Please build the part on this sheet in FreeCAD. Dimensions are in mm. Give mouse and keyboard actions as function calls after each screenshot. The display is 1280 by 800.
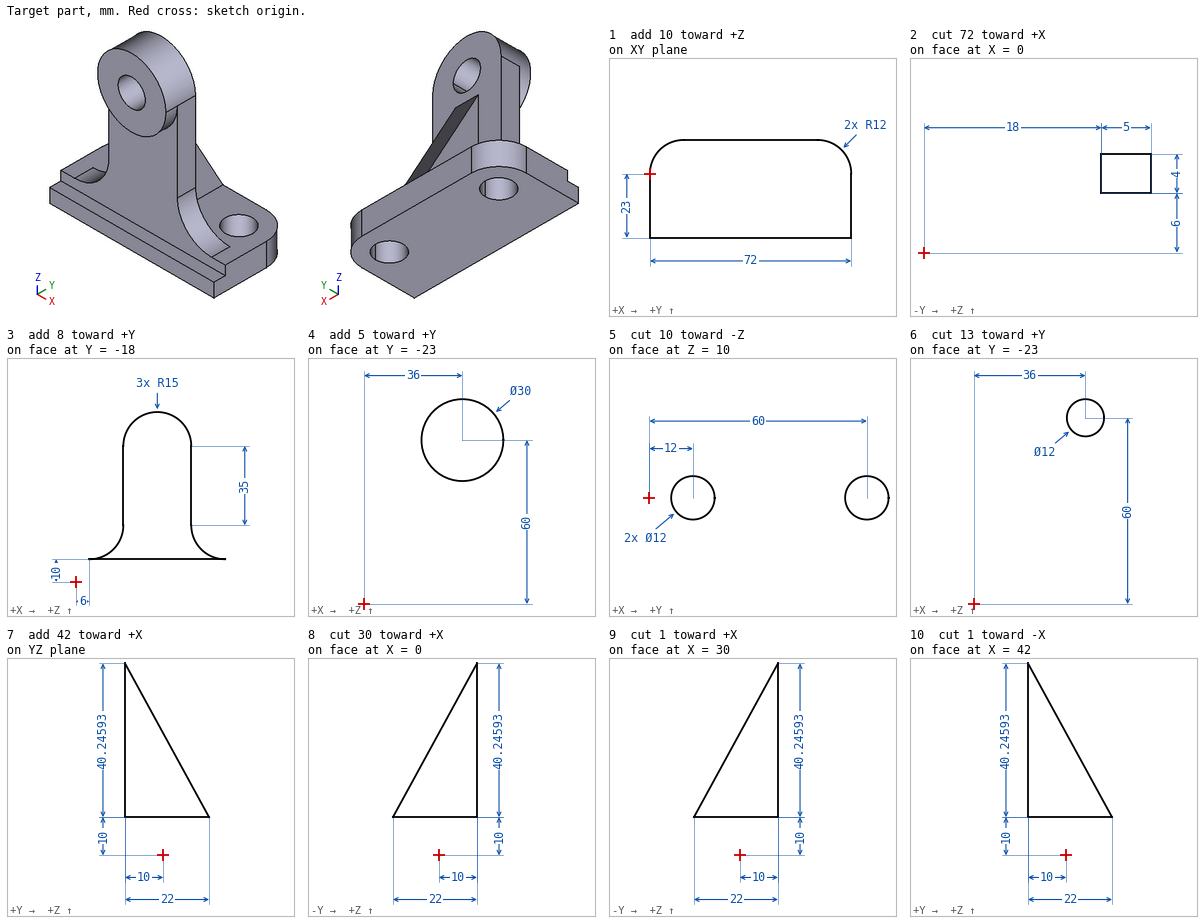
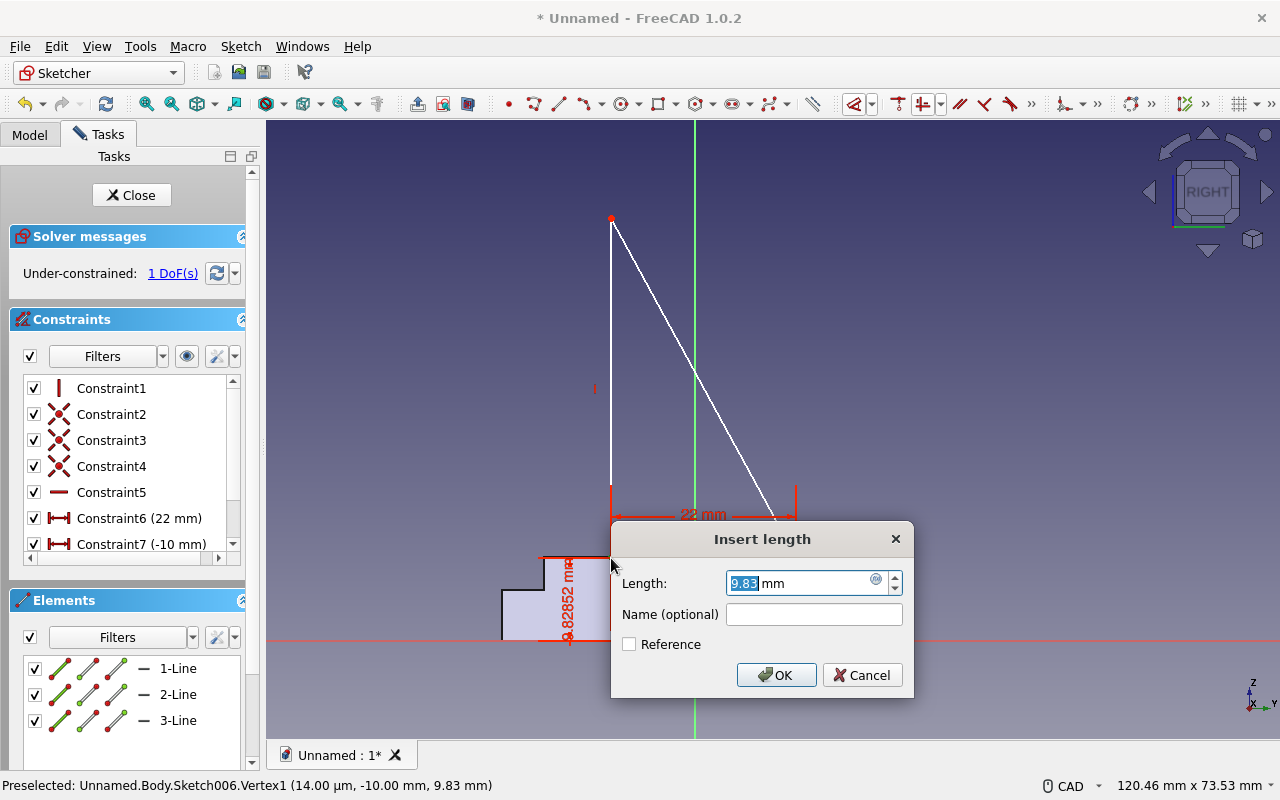
text(10)
key(Return)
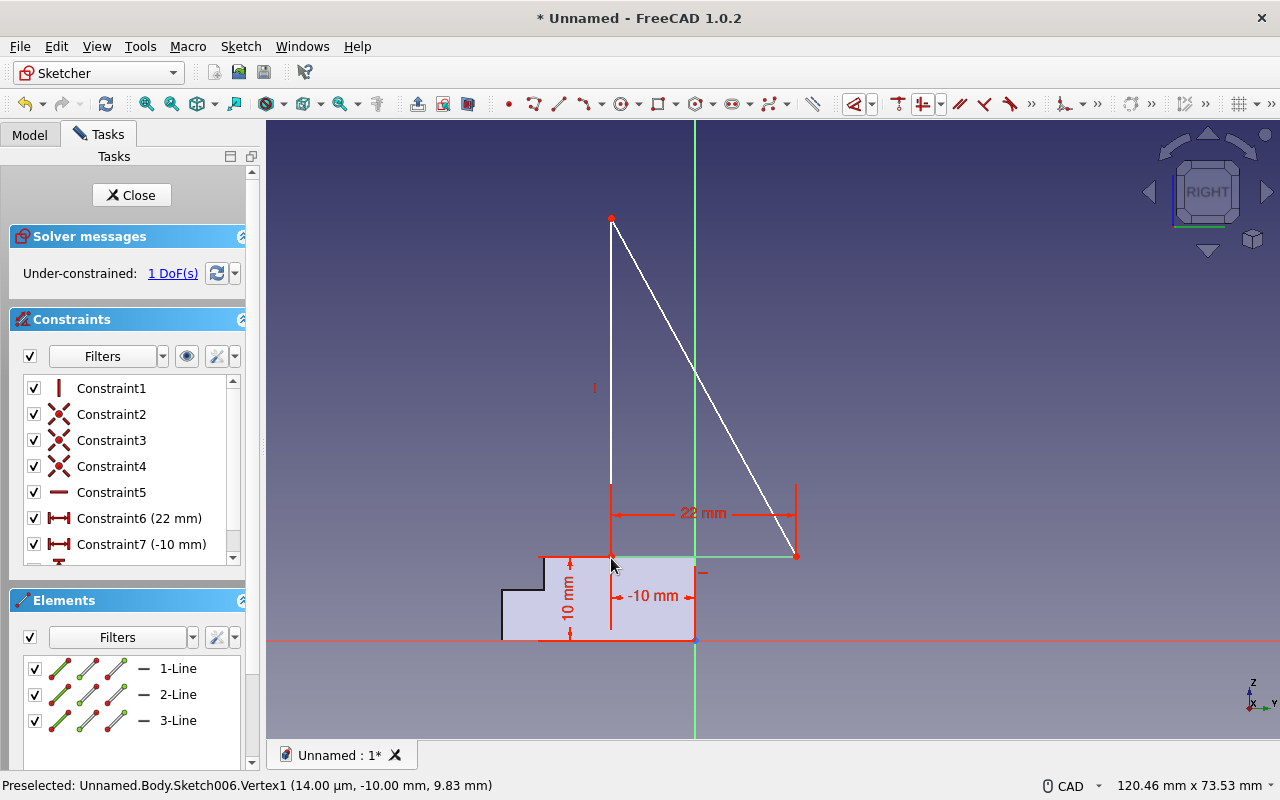
click(611, 455)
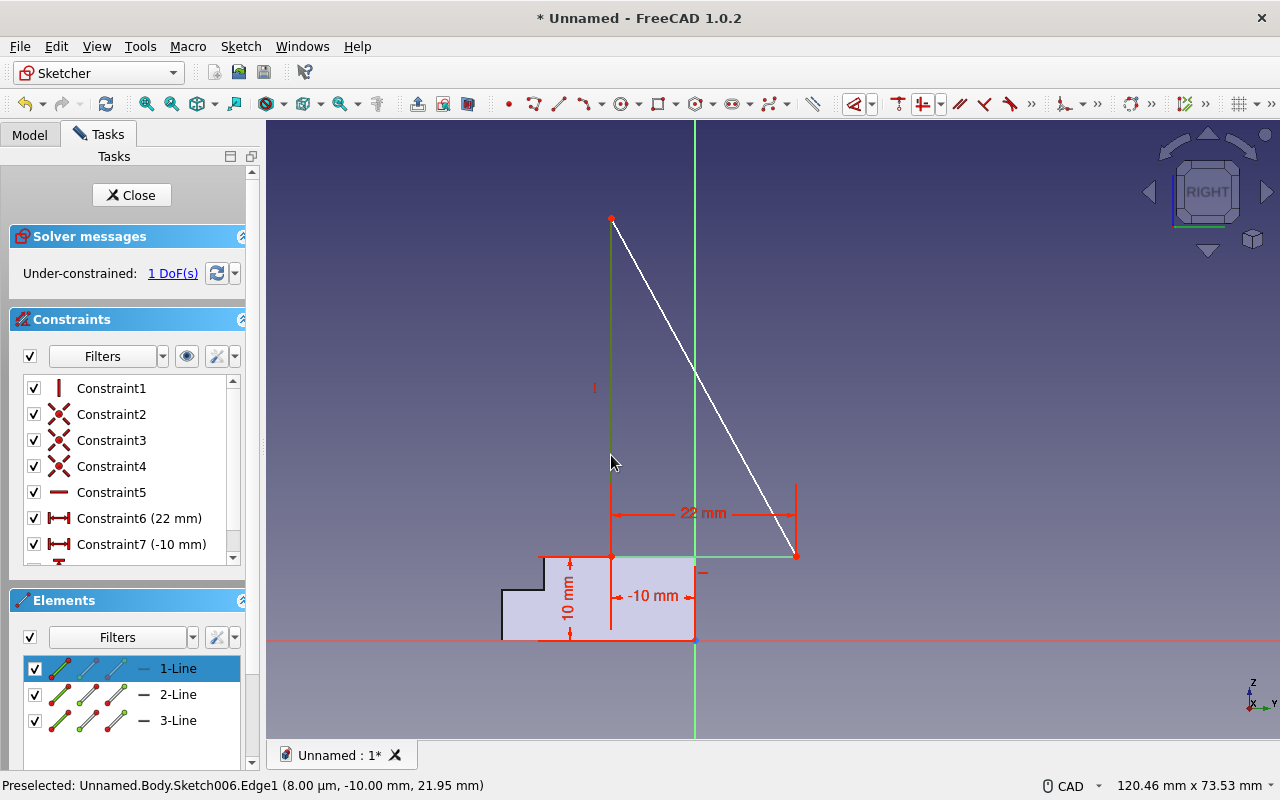
key(i)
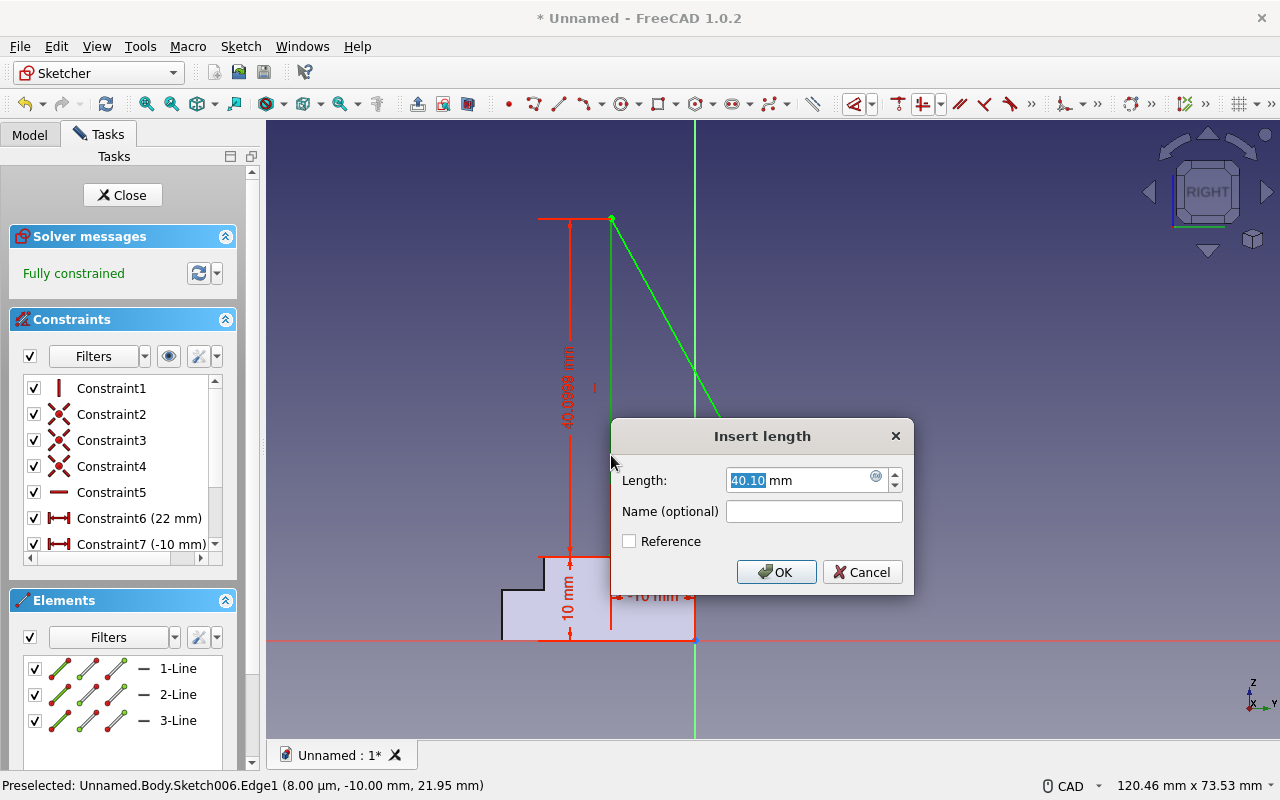
text(40.24593)
key(Return)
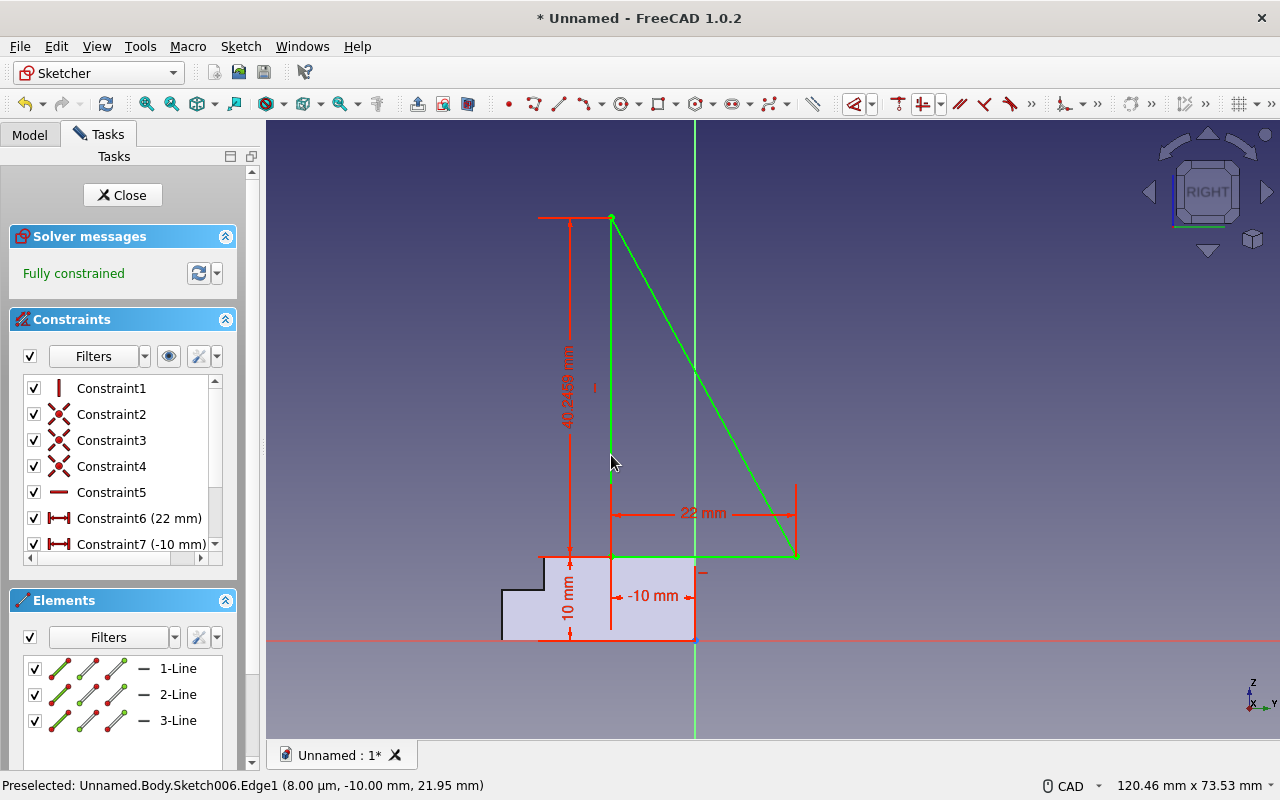
click(123, 195)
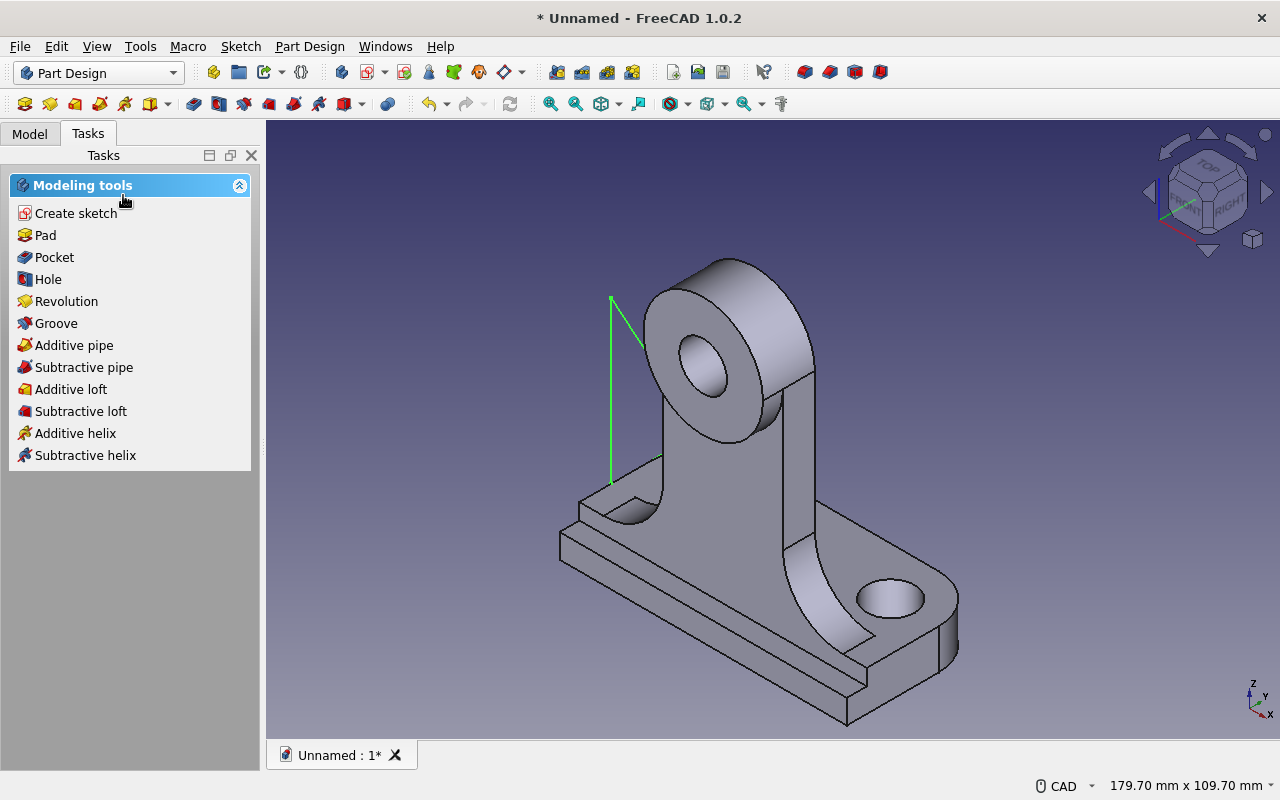
click(25, 104)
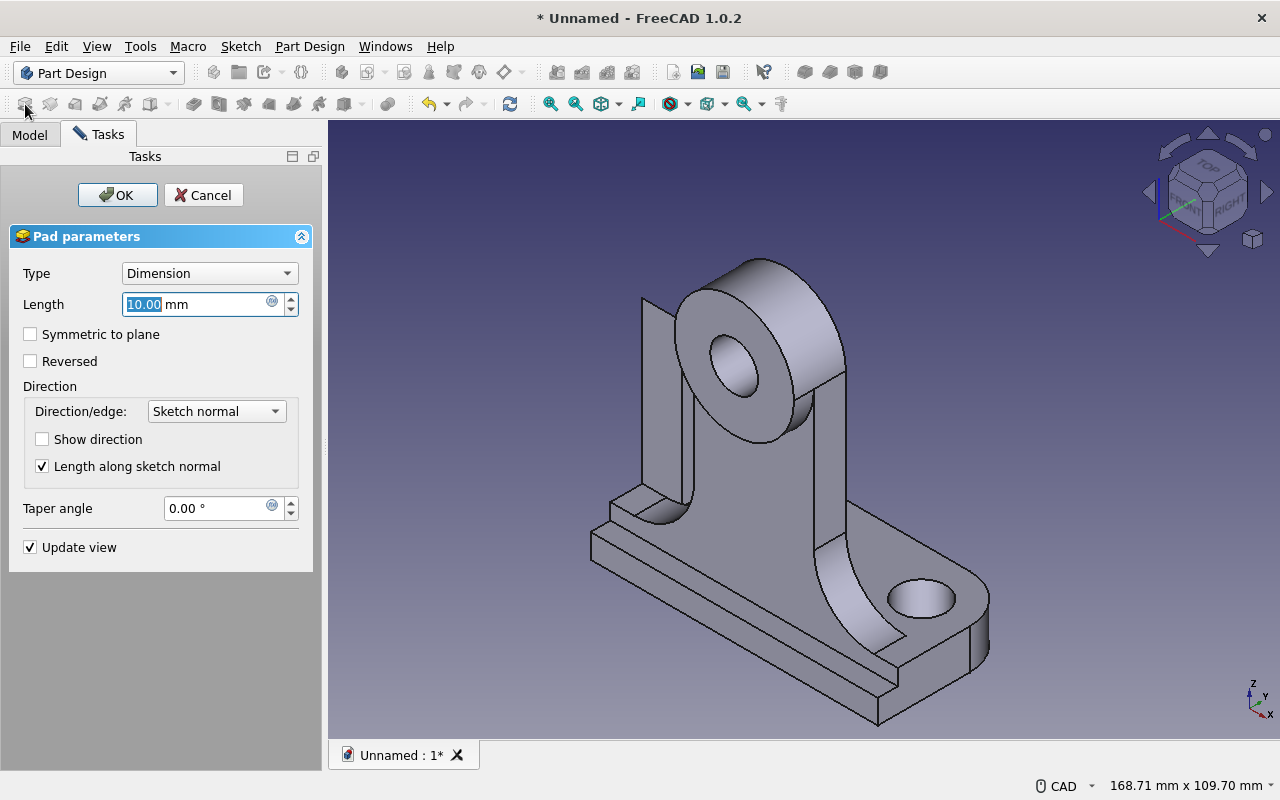
text(42)
key(Tab)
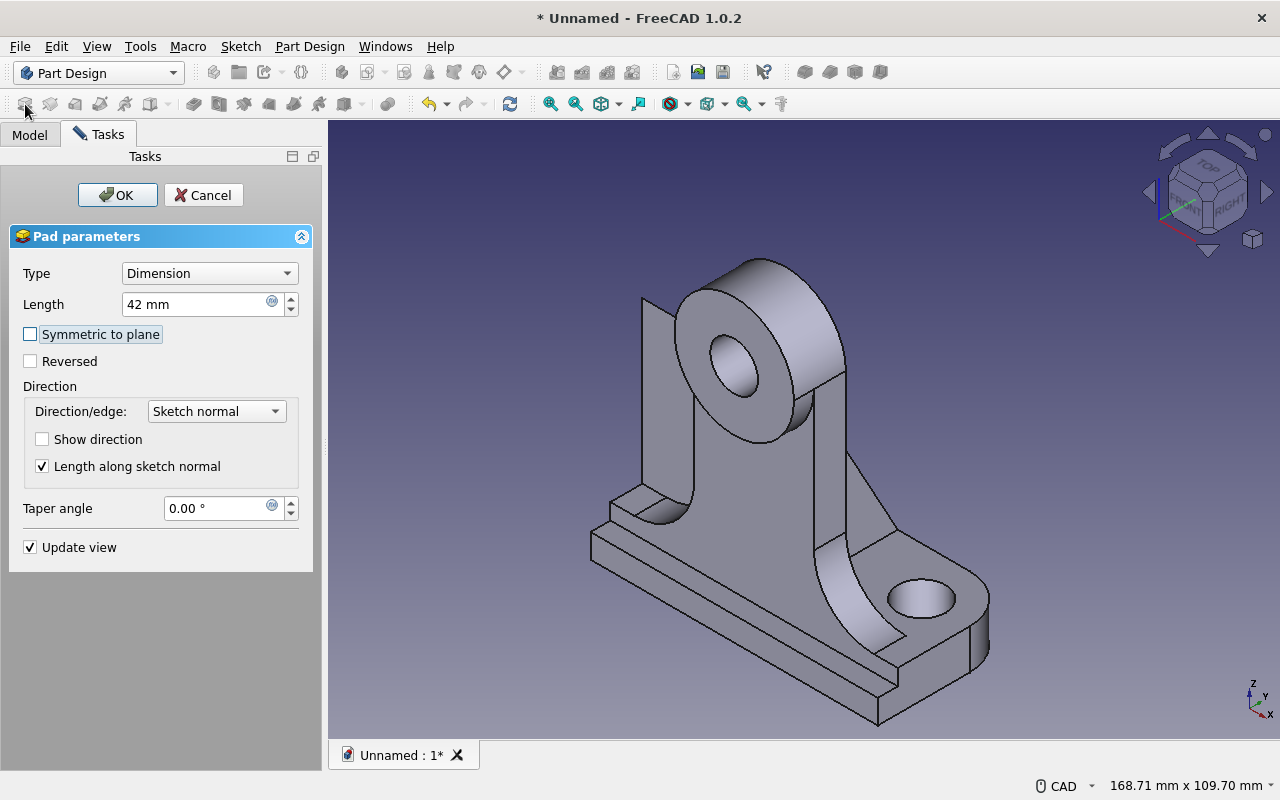
click(118, 195)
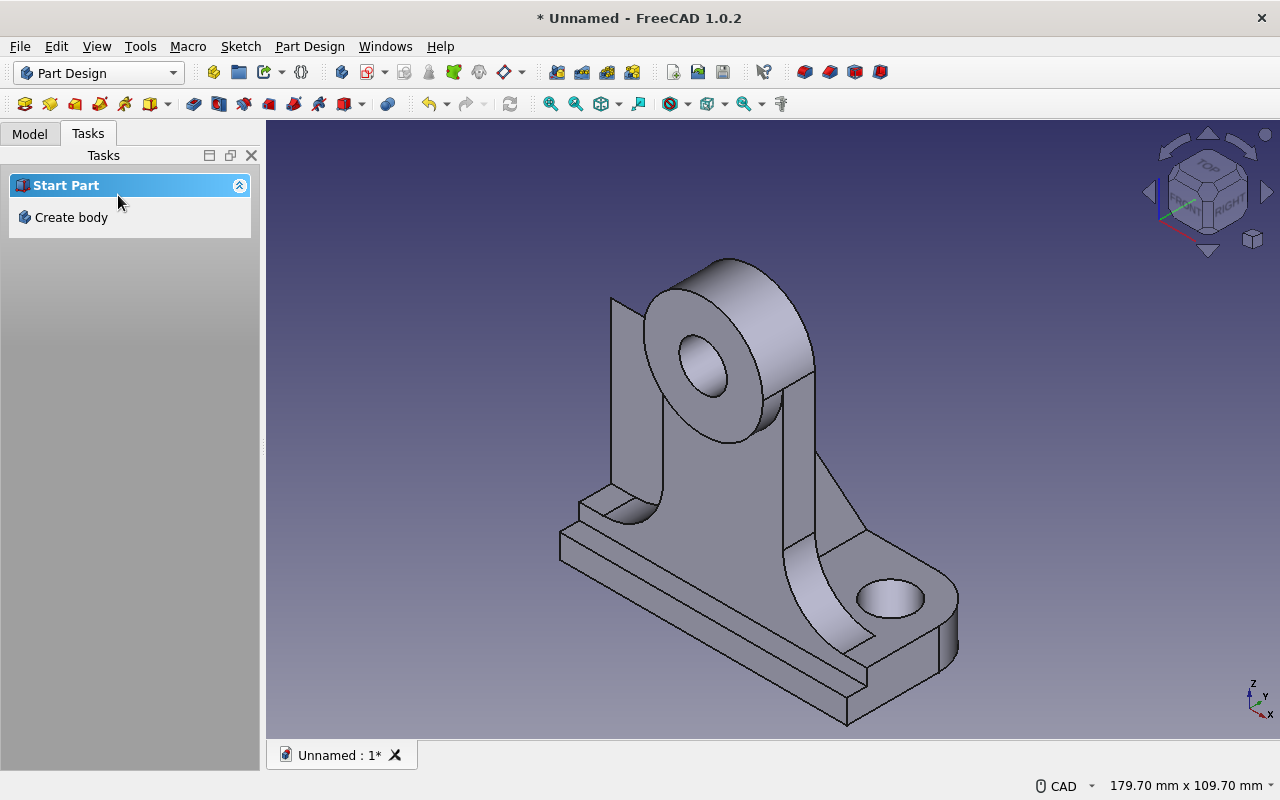
key(6)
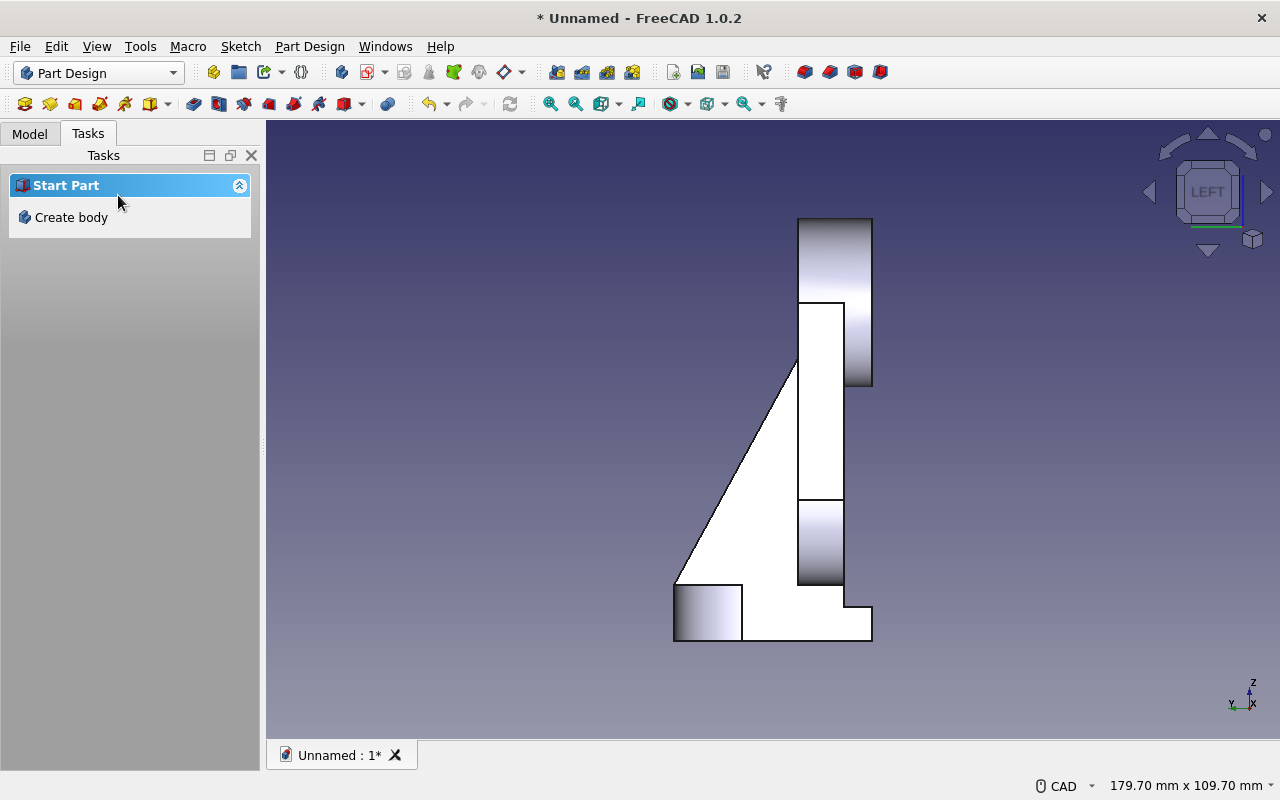
click(745, 539)